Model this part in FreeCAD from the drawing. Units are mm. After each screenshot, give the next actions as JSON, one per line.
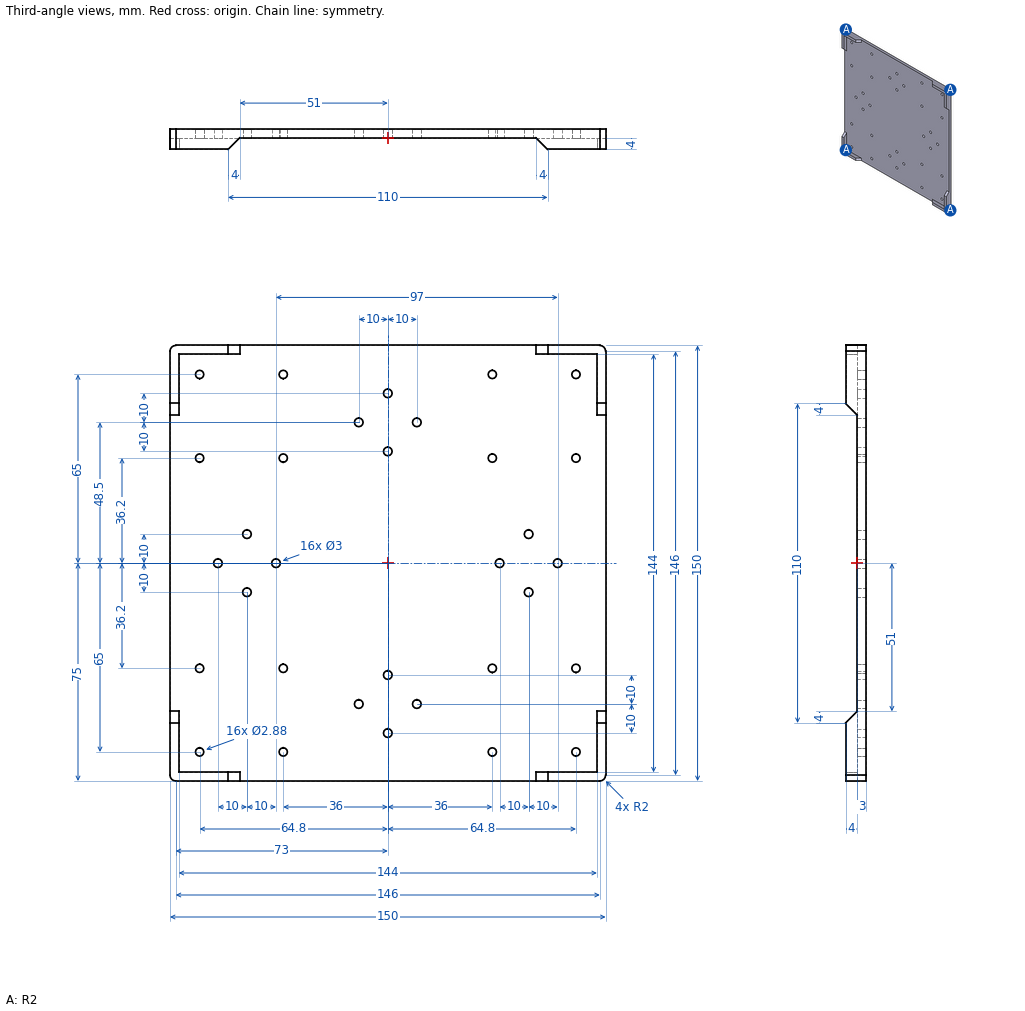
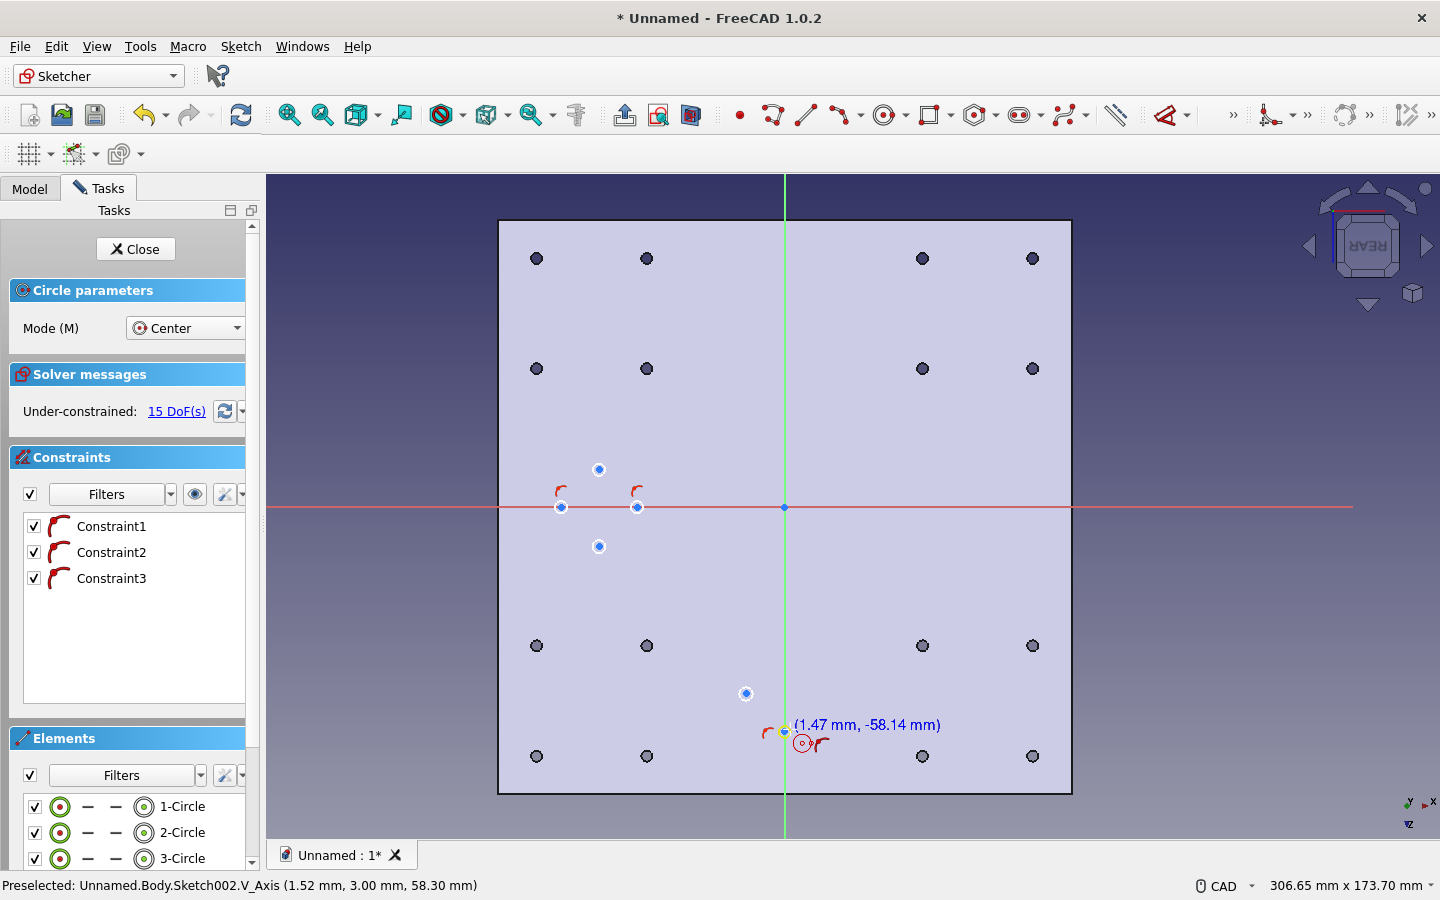
{"action": "left_click", "coordinate": [823, 693]}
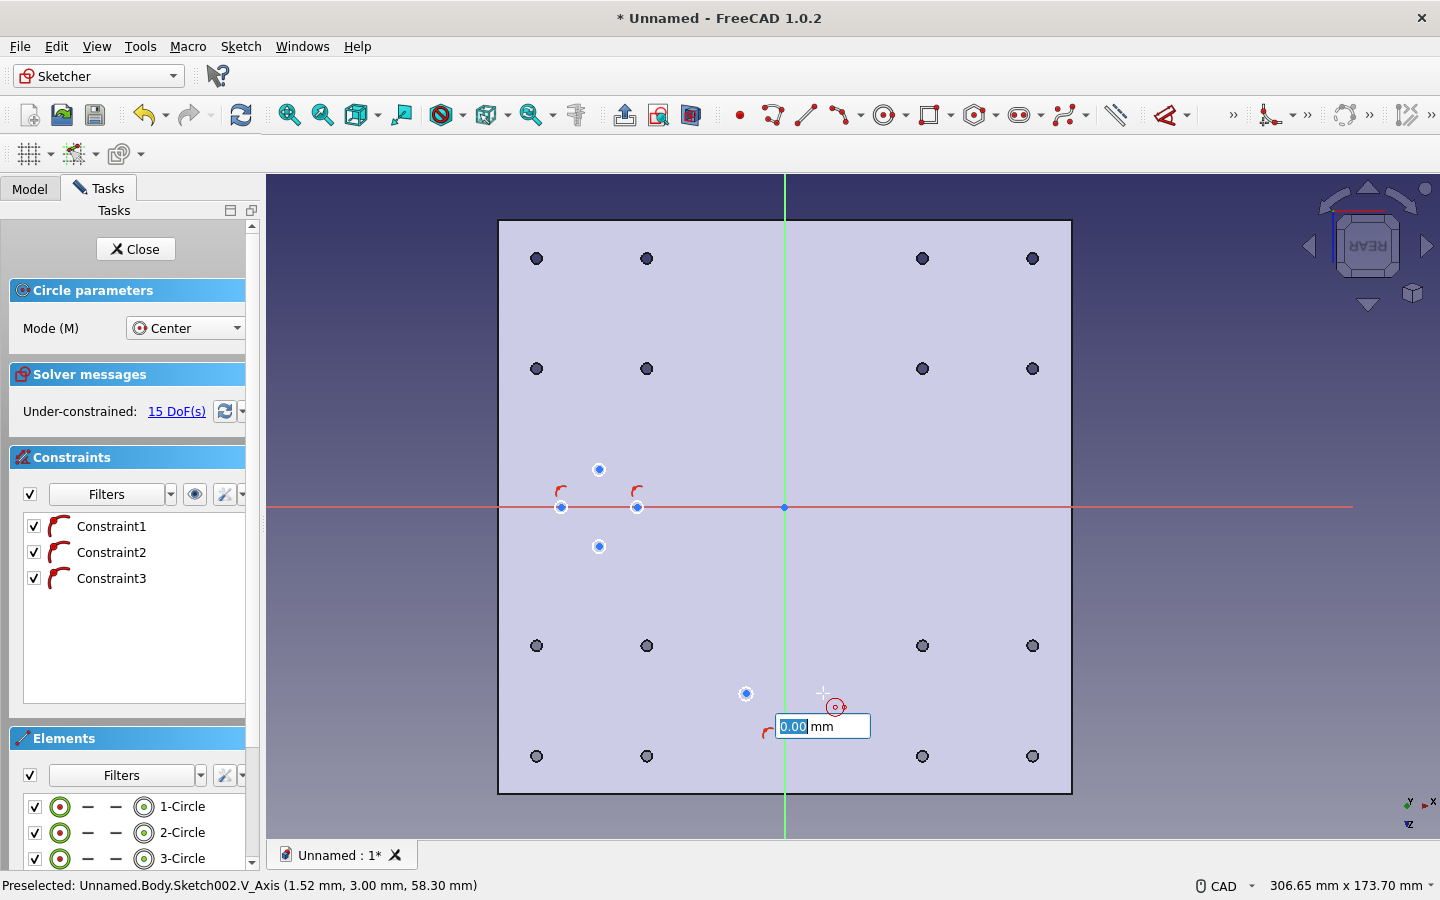
{"action": "scroll", "coordinate": [827, 689], "scroll_direction": "up", "scroll_amount": 6}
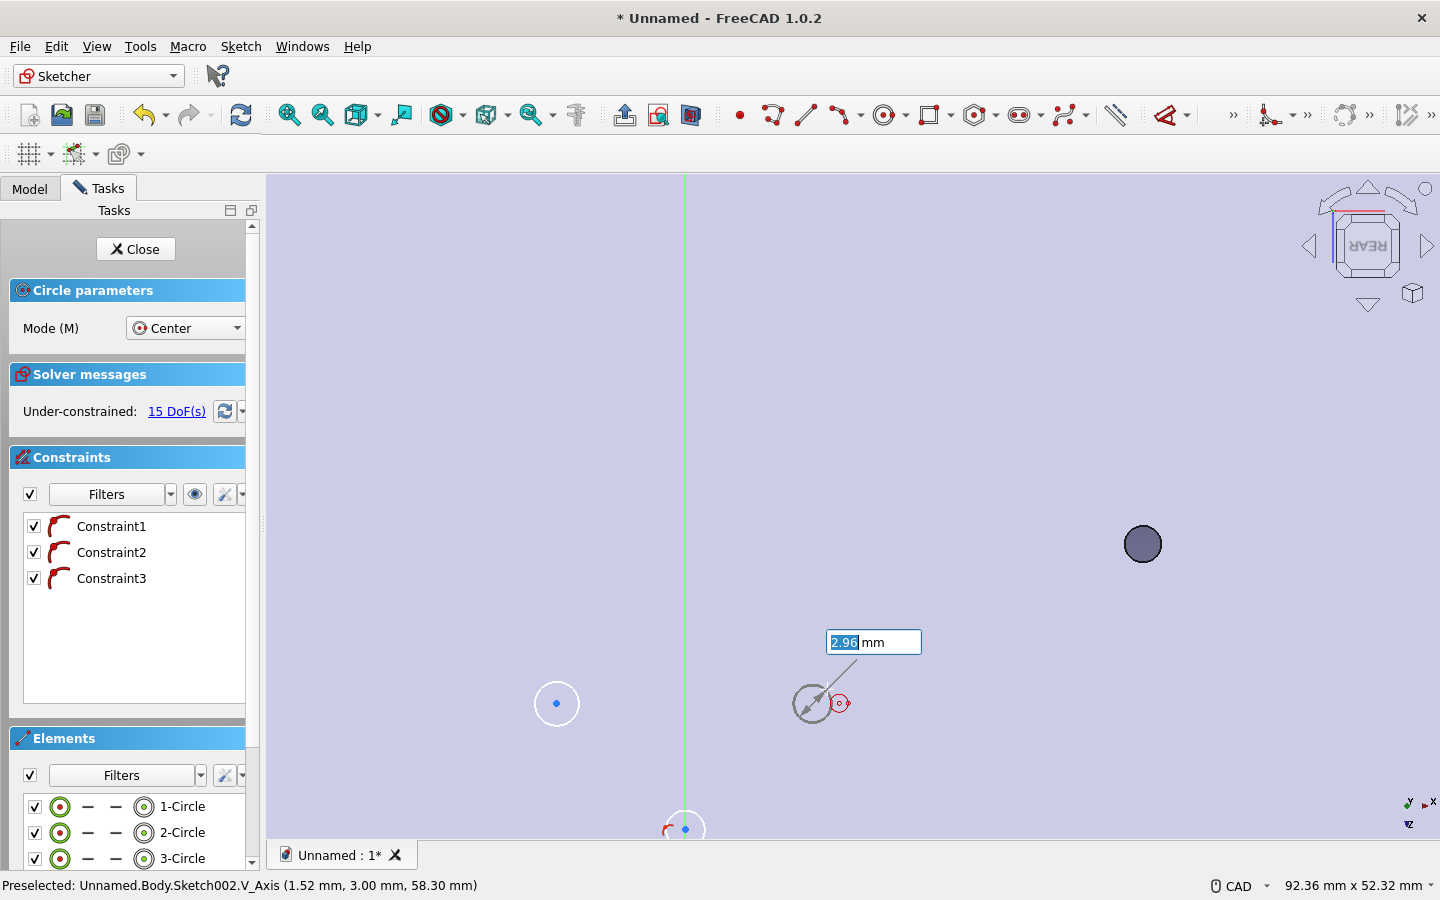
{"action": "left_click", "coordinate": [826, 687]}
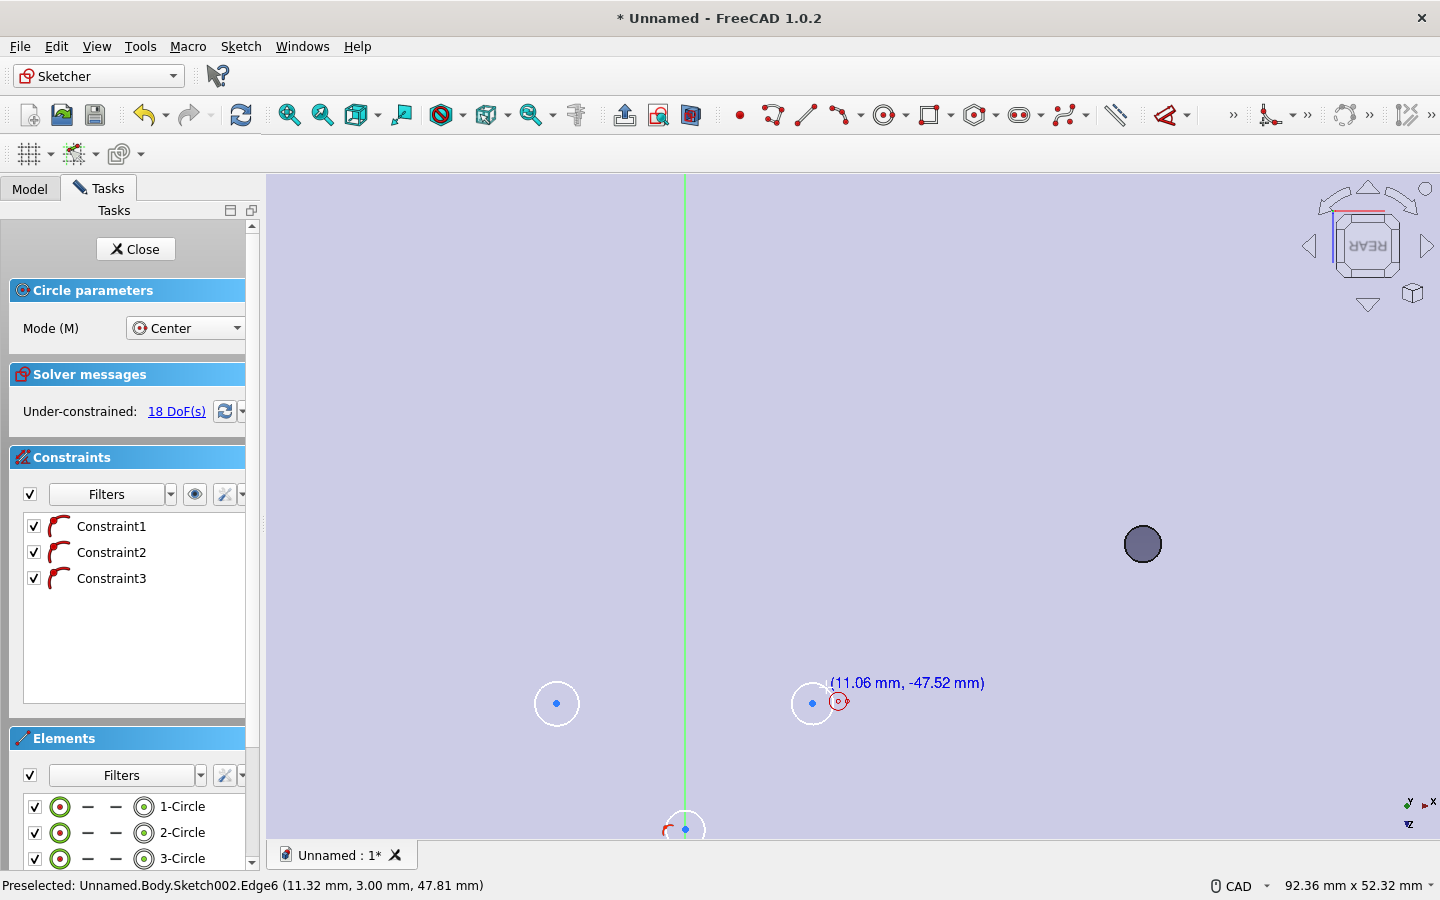
{"action": "scroll", "coordinate": [827, 689], "scroll_direction": "down", "scroll_amount": 6}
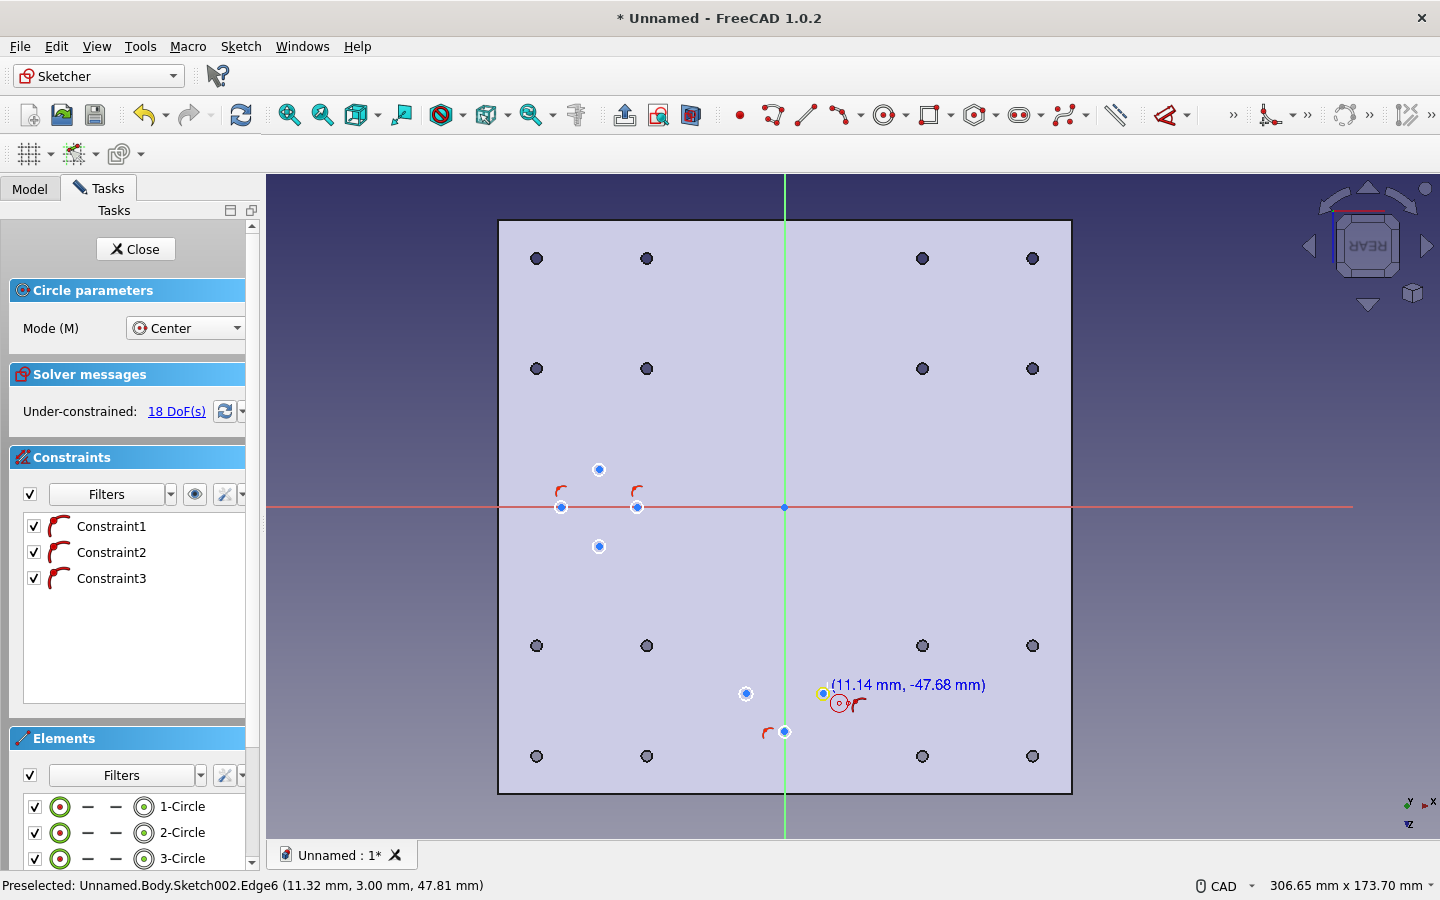
{"action": "left_click", "coordinate": [785, 655]}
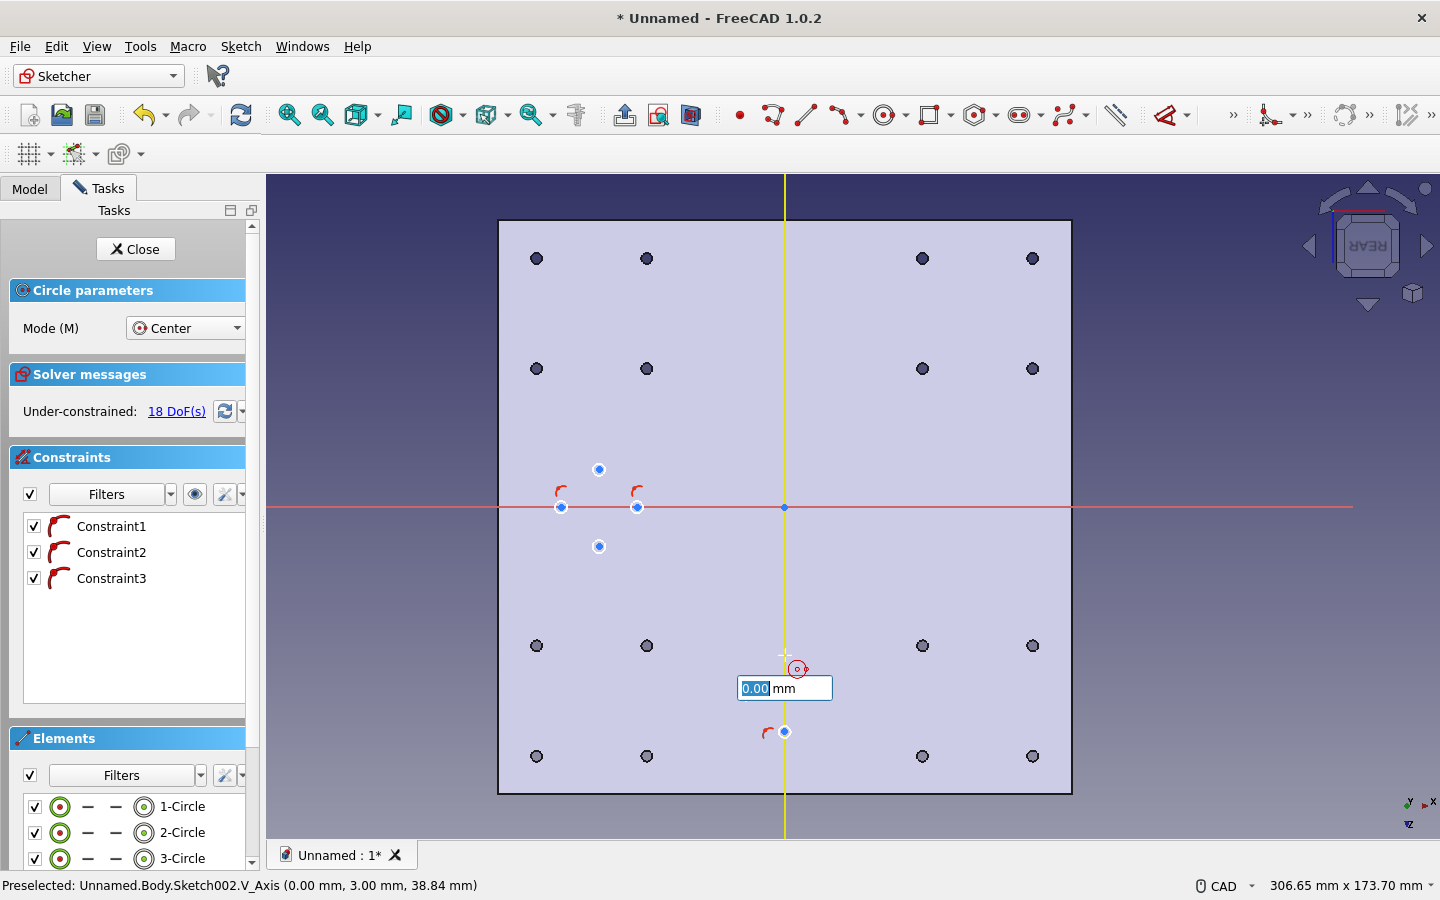
{"action": "scroll", "coordinate": [790, 653], "scroll_direction": "up", "scroll_amount": 6}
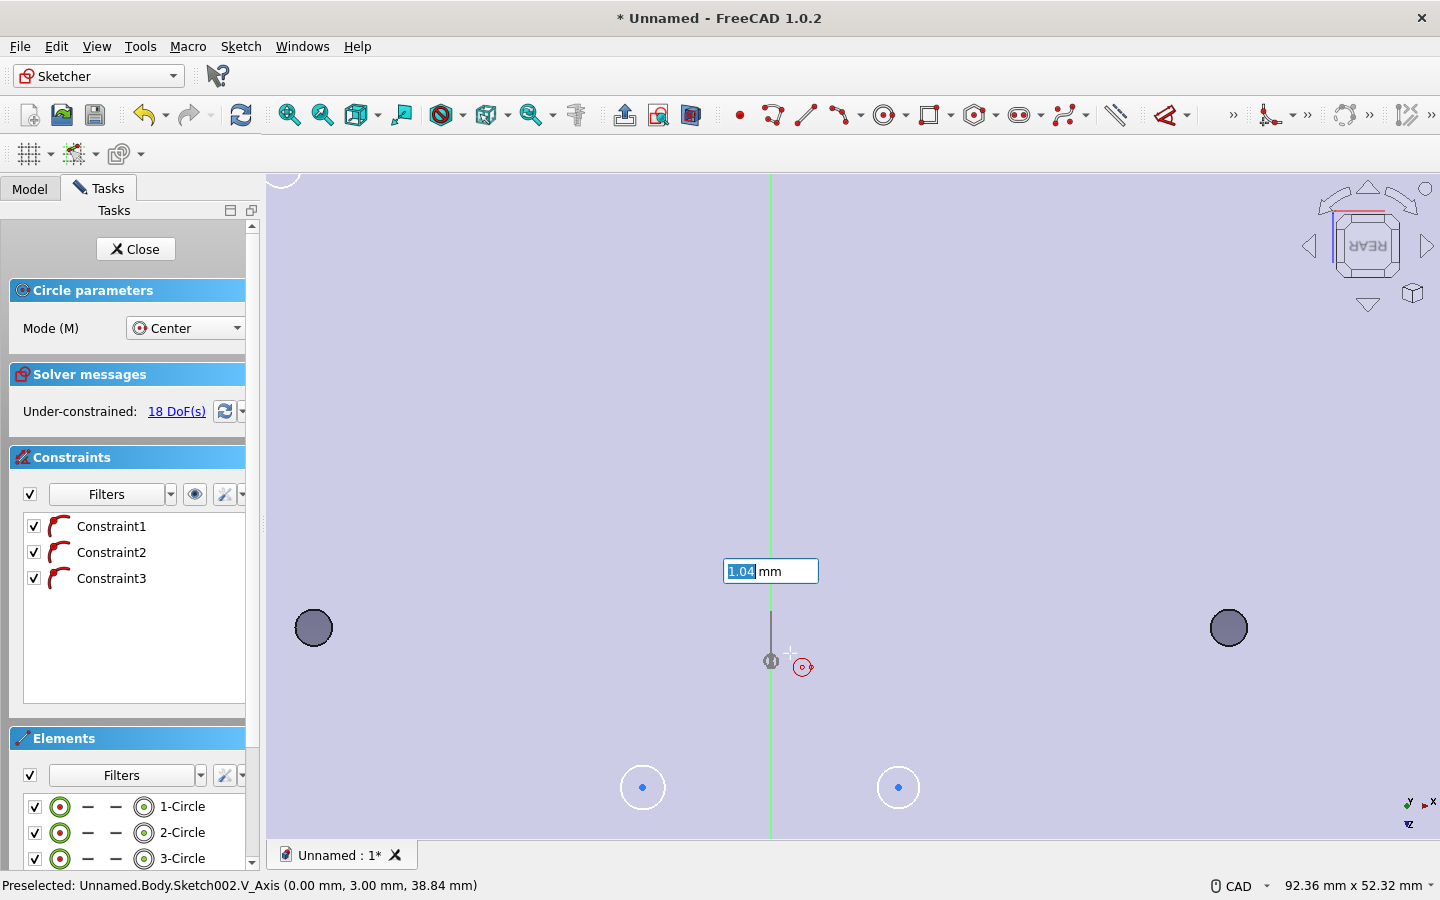
{"action": "left_click", "coordinate": [789, 650]}